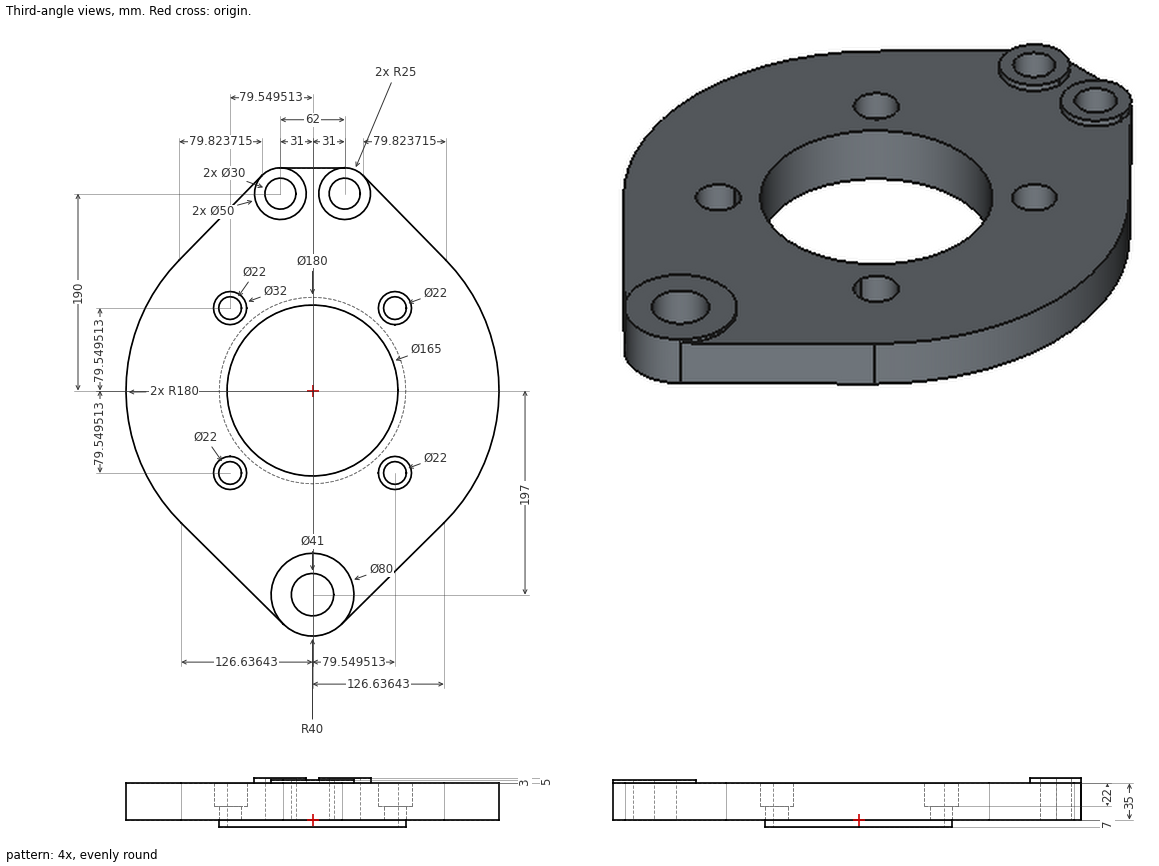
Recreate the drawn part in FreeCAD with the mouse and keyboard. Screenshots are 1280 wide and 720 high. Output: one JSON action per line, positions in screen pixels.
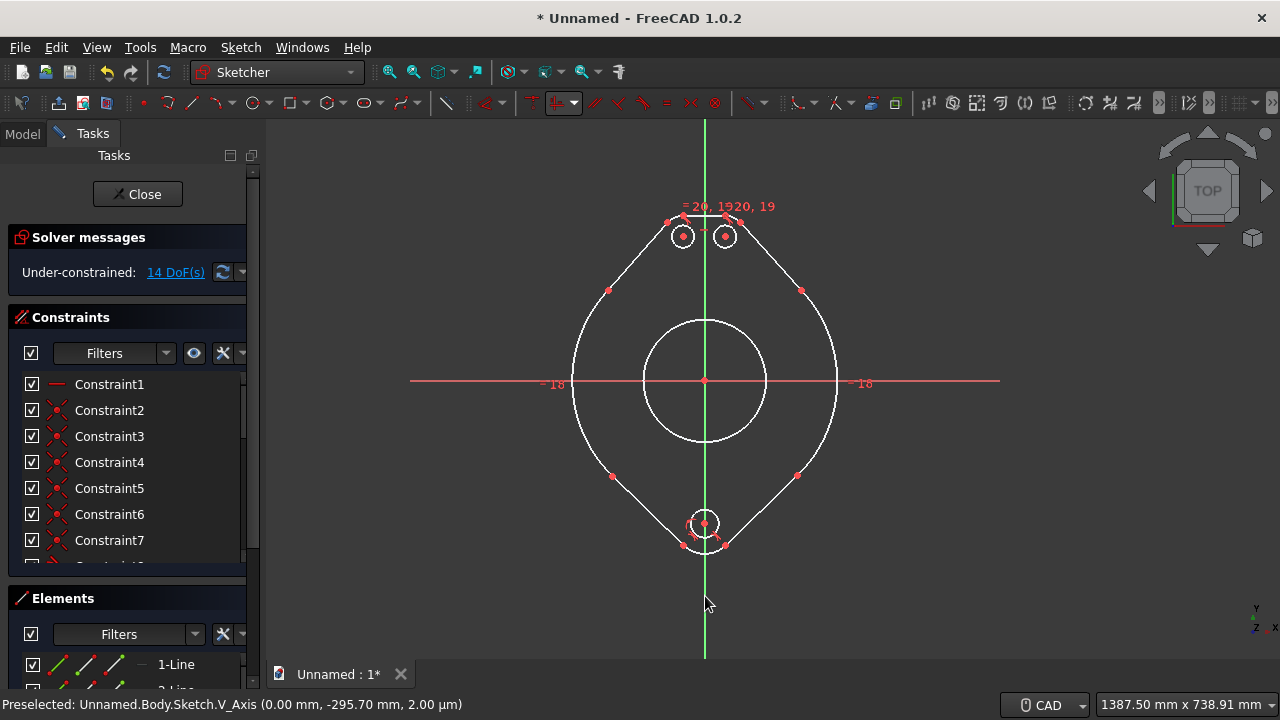
{"action": "left_click", "coordinate": [578, 343]}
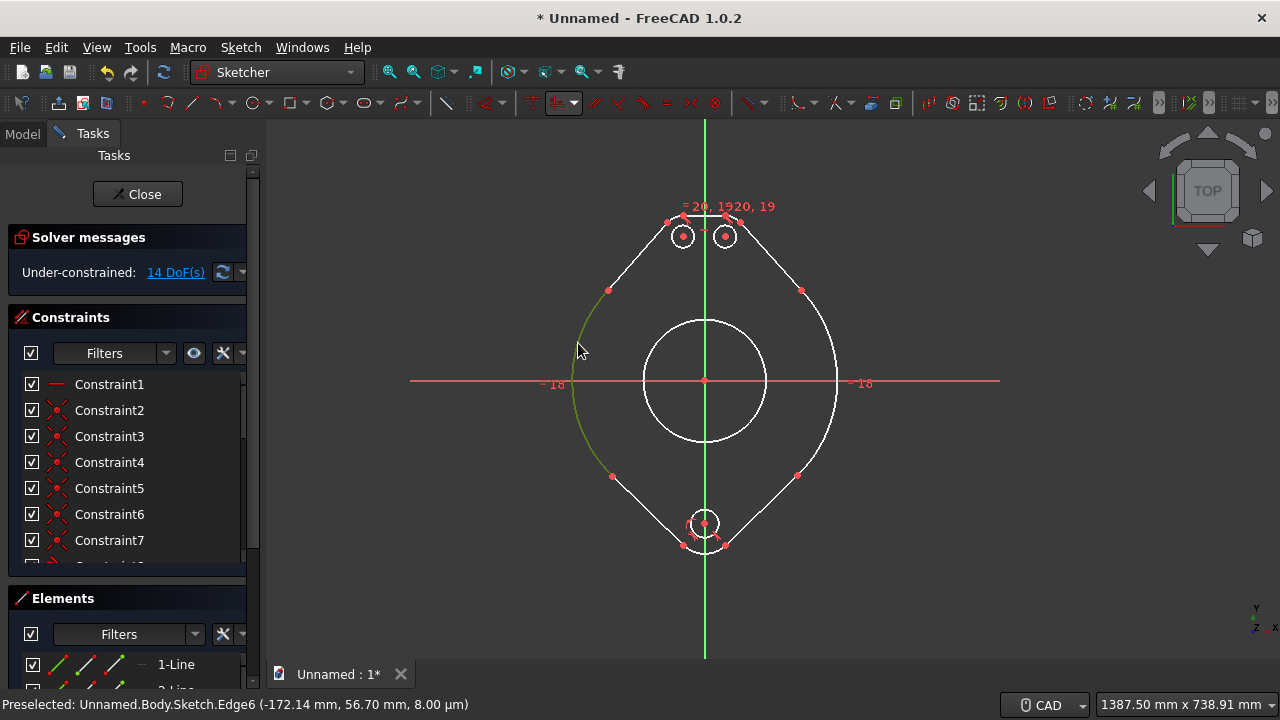
{"action": "key", "text": "k r"}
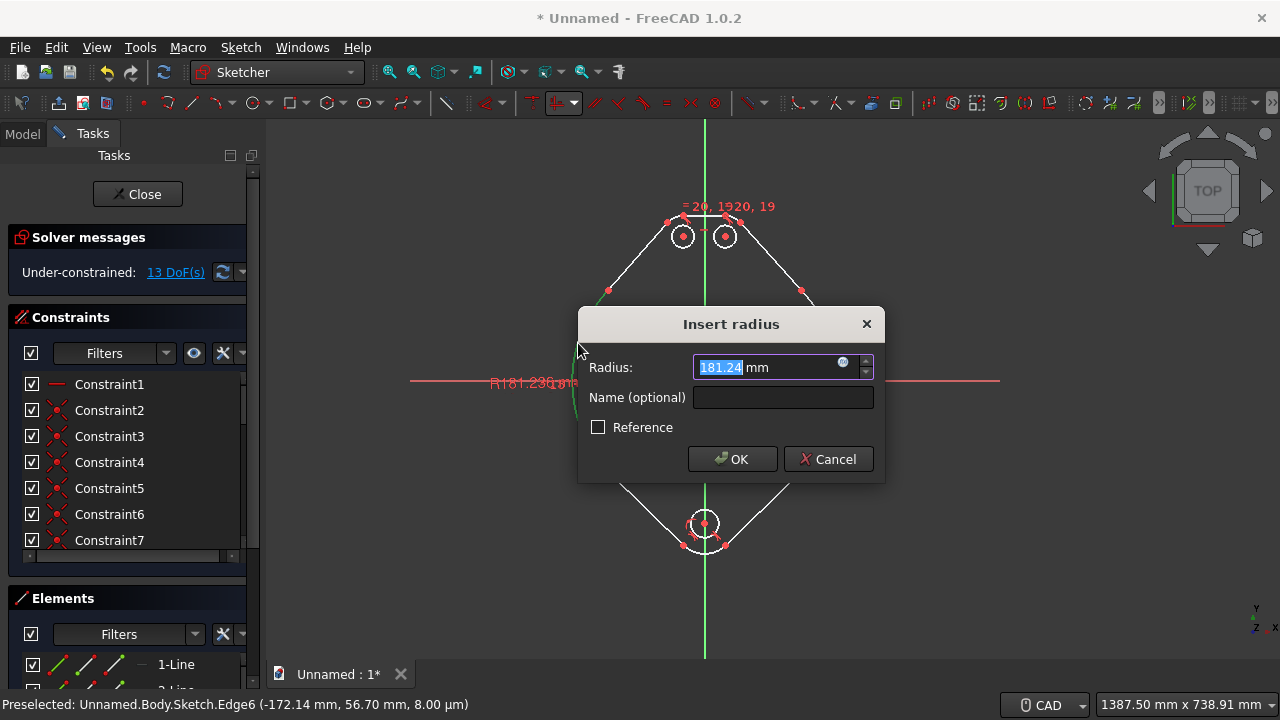
{"action": "type", "text": "180"}
{"action": "key", "text": "Return"}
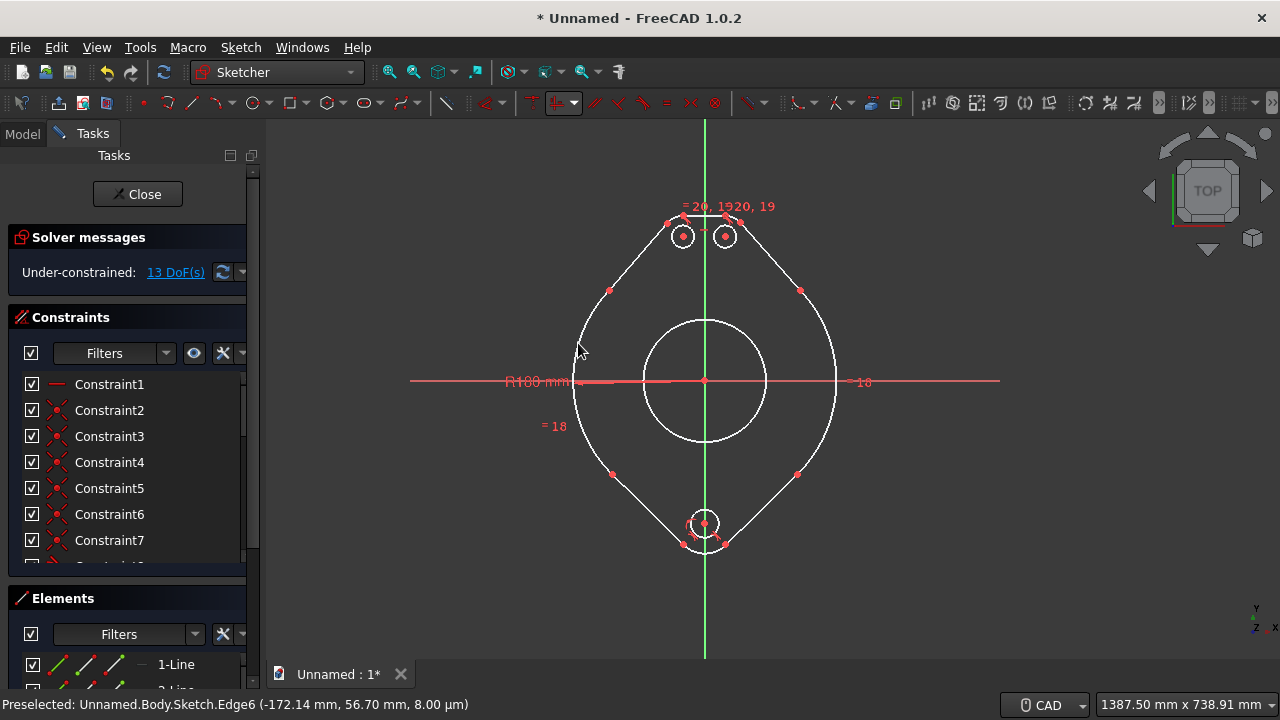
{"action": "scroll", "coordinate": [696, 552], "scroll_direction": "up", "scroll_amount": 3}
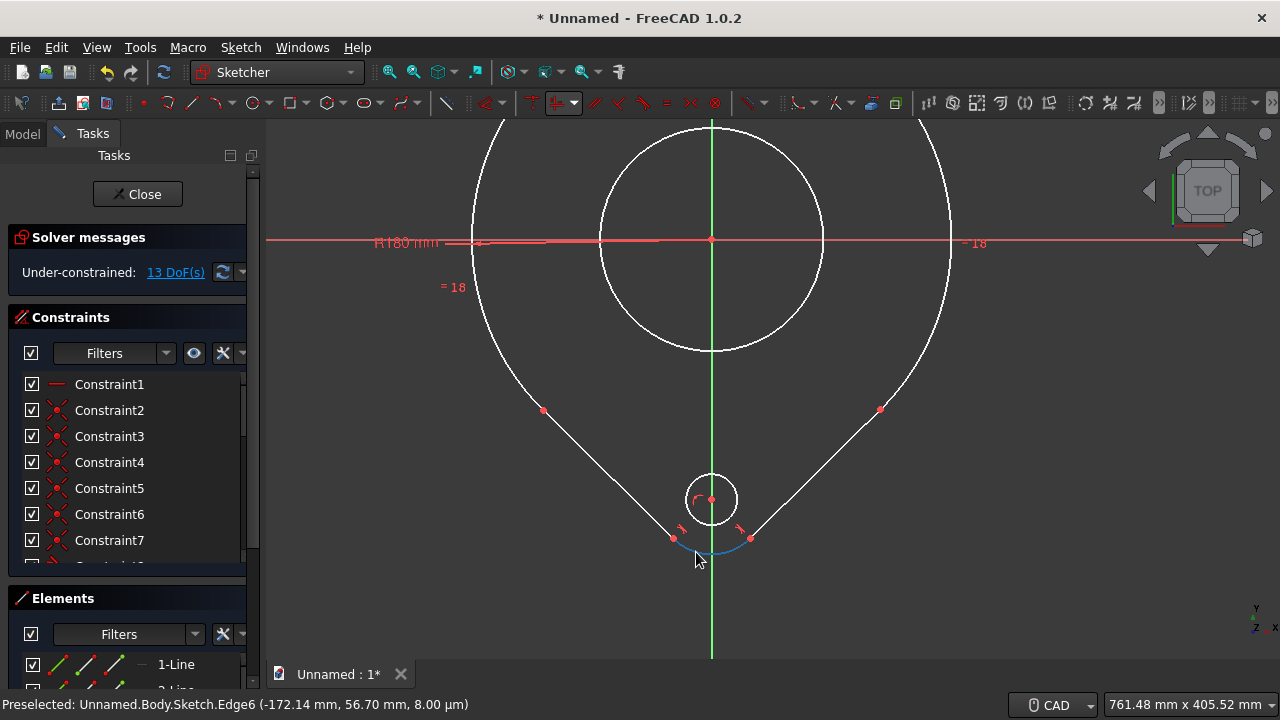
{"action": "left_click", "coordinate": [695, 552]}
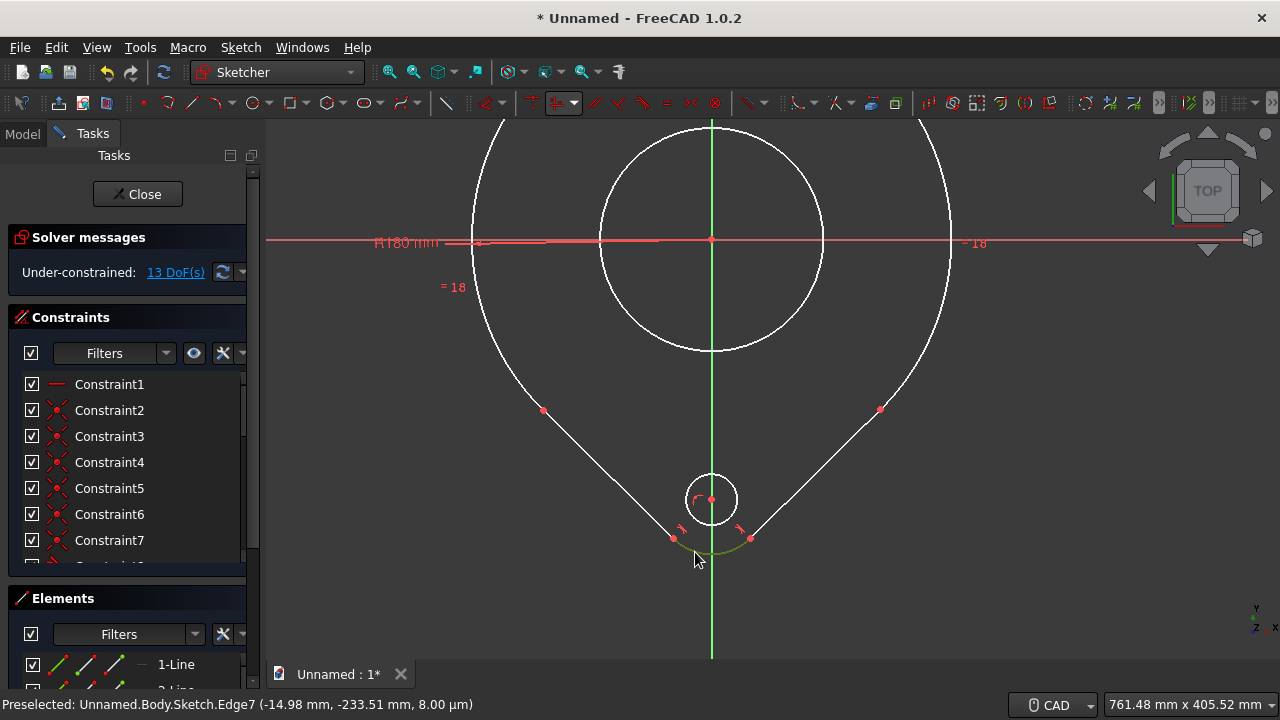
{"action": "key", "text": "k r"}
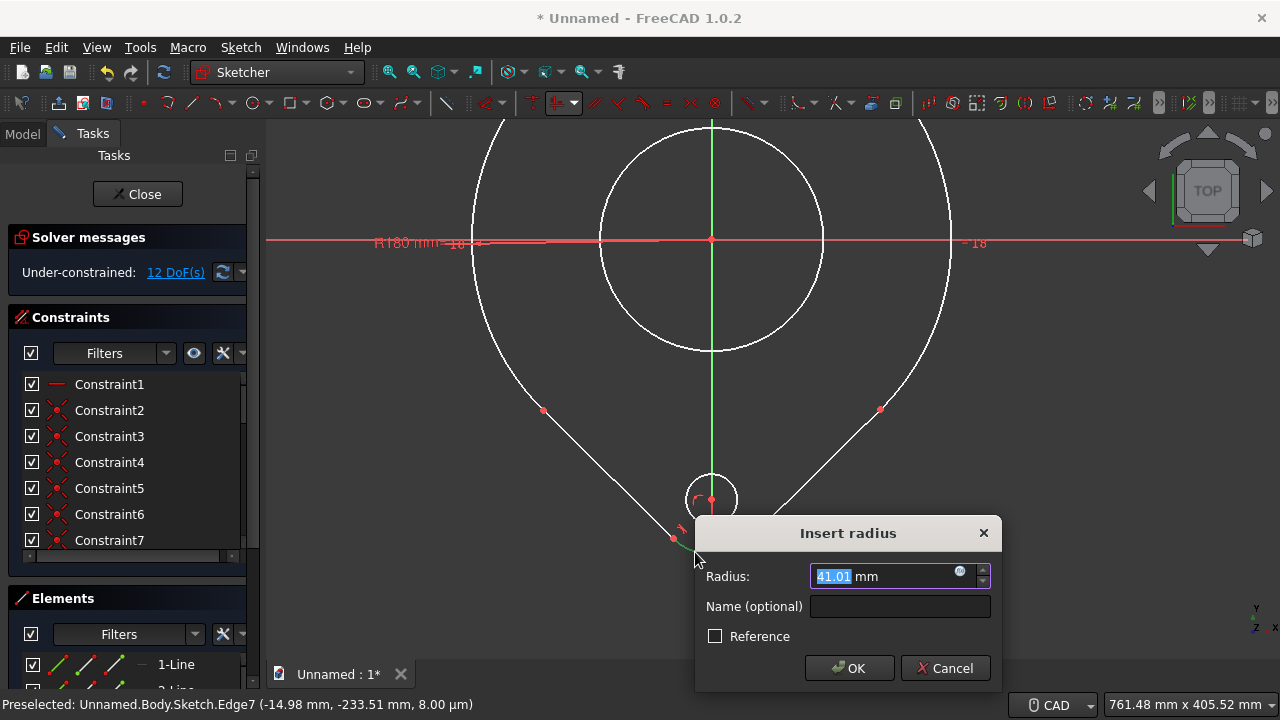
{"action": "type", "text": "40"}
{"action": "key", "text": "Return"}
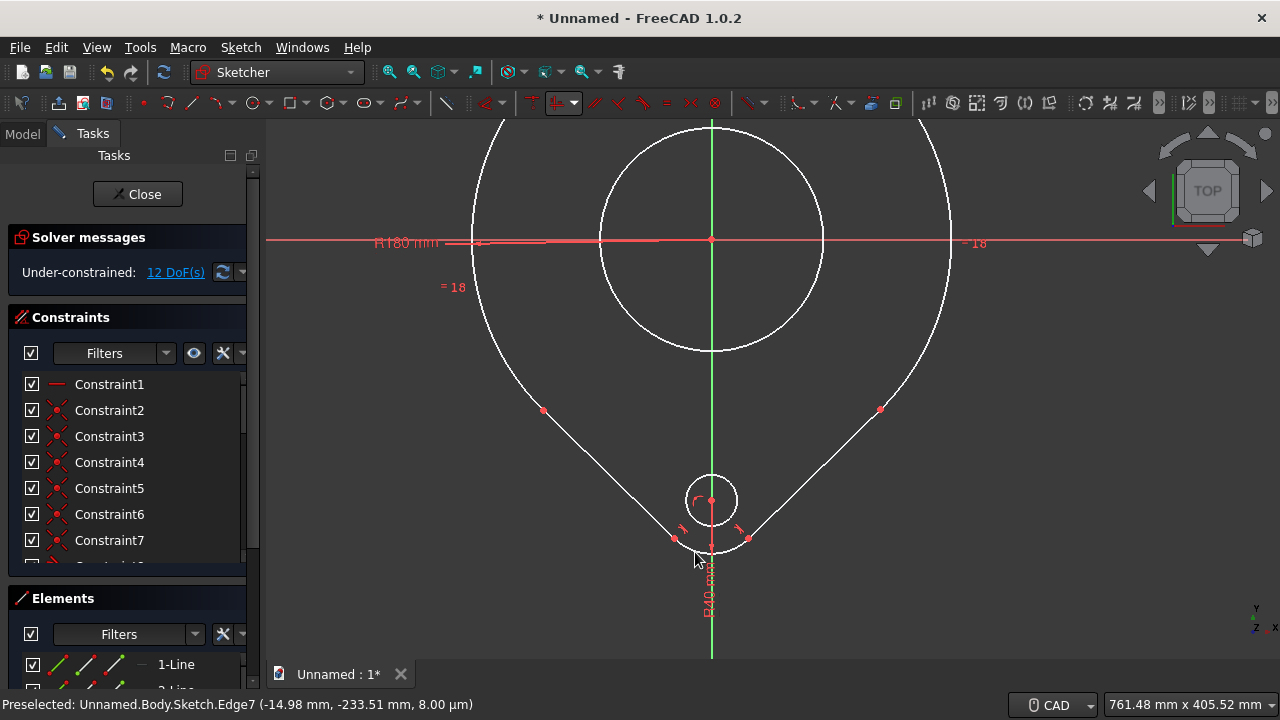
{"action": "scroll", "coordinate": [696, 553], "scroll_direction": "down", "scroll_amount": 3}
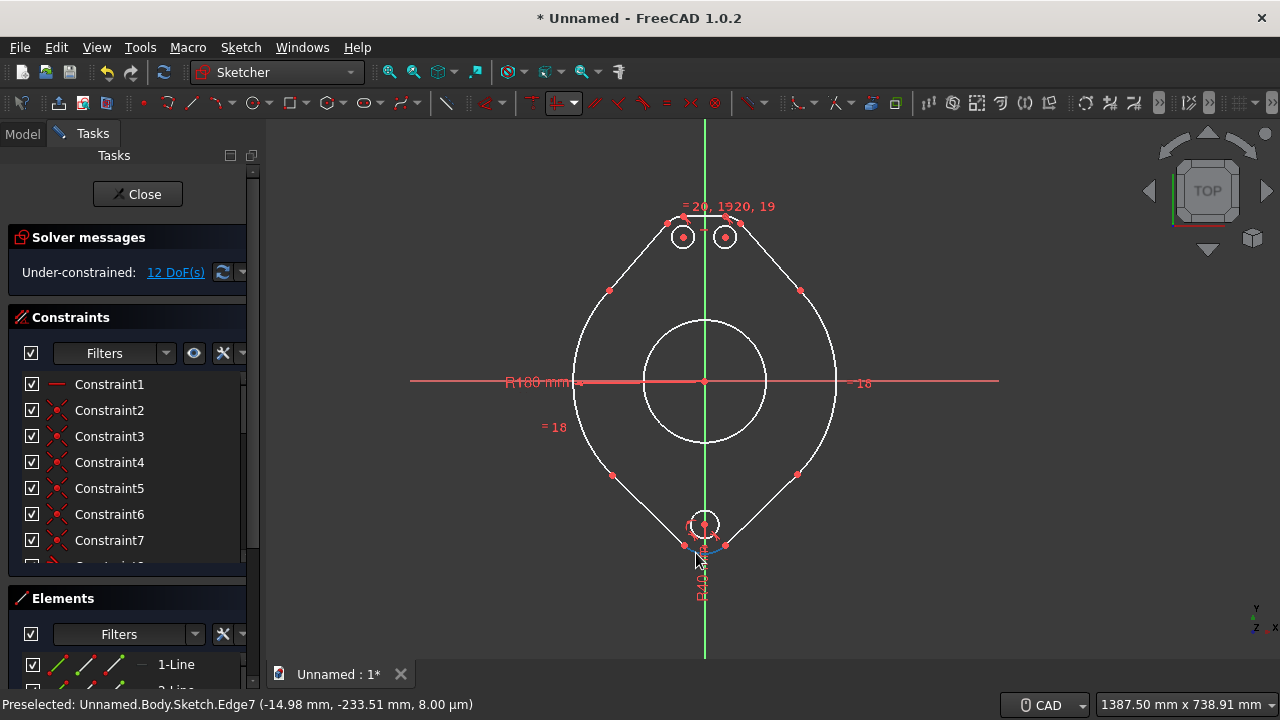
{"action": "scroll", "coordinate": [737, 220], "scroll_direction": "up", "scroll_amount": 5}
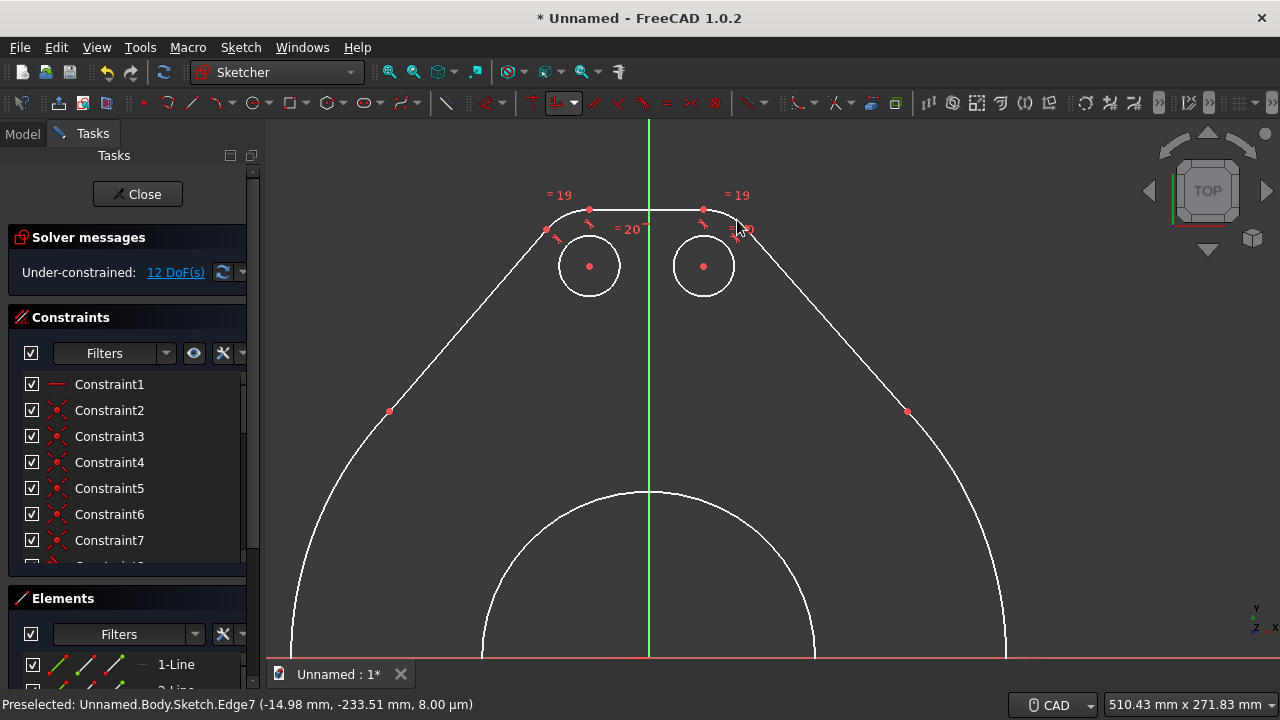
{"action": "left_click", "coordinate": [735, 219]}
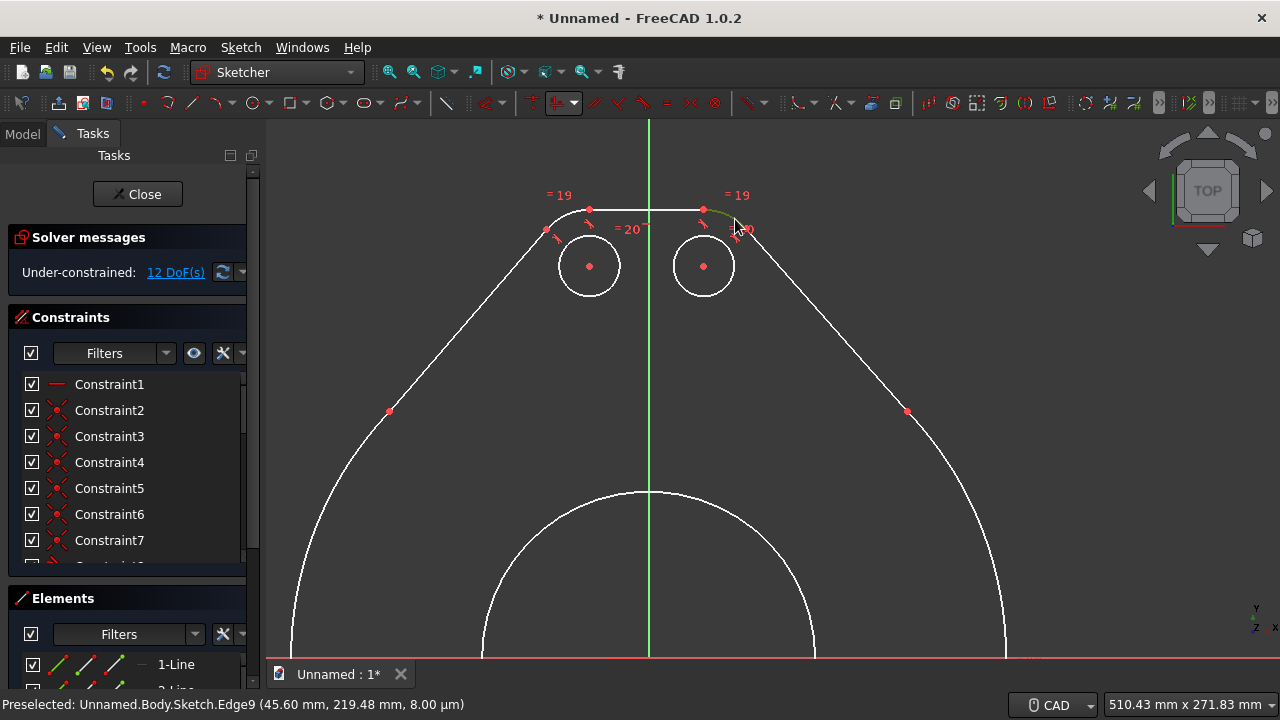
{"action": "left_click", "coordinate": [504, 104]}